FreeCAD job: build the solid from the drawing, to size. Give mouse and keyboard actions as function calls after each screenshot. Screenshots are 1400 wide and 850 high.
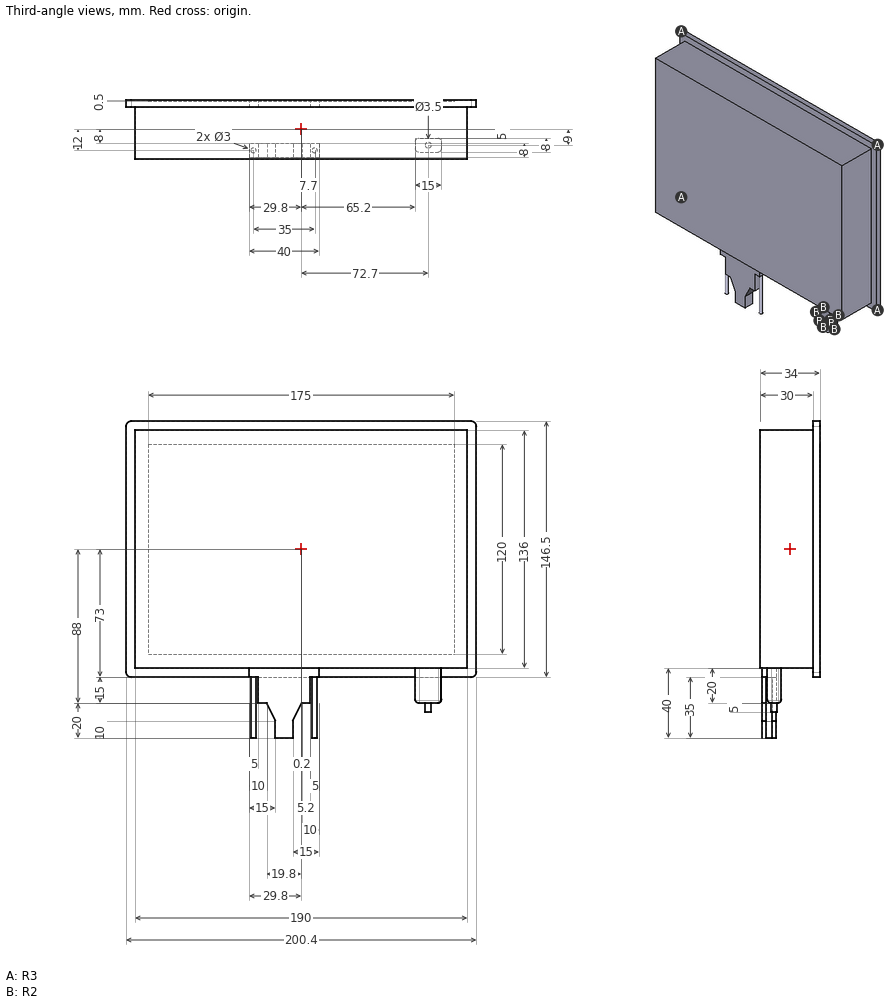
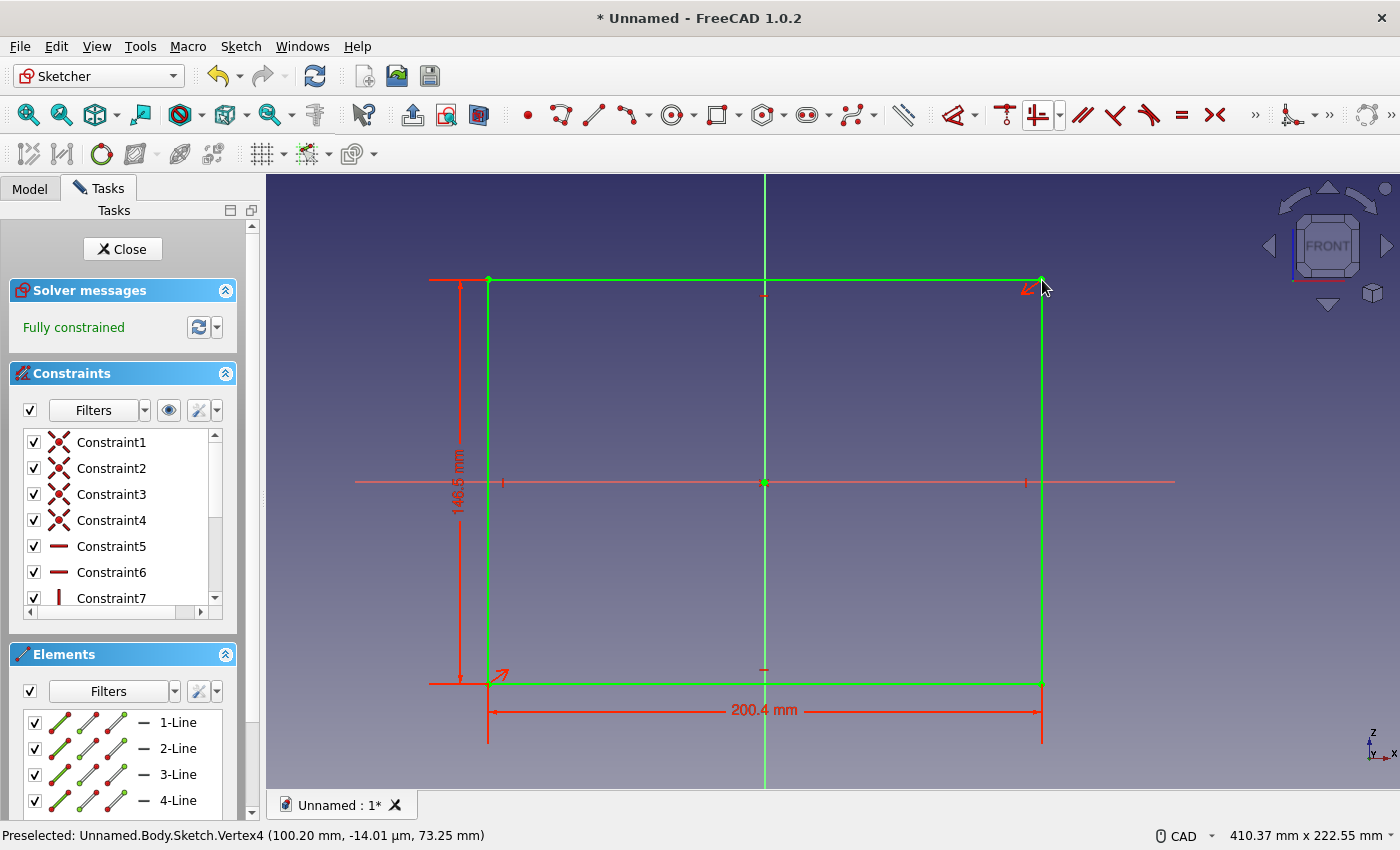
click(123, 249)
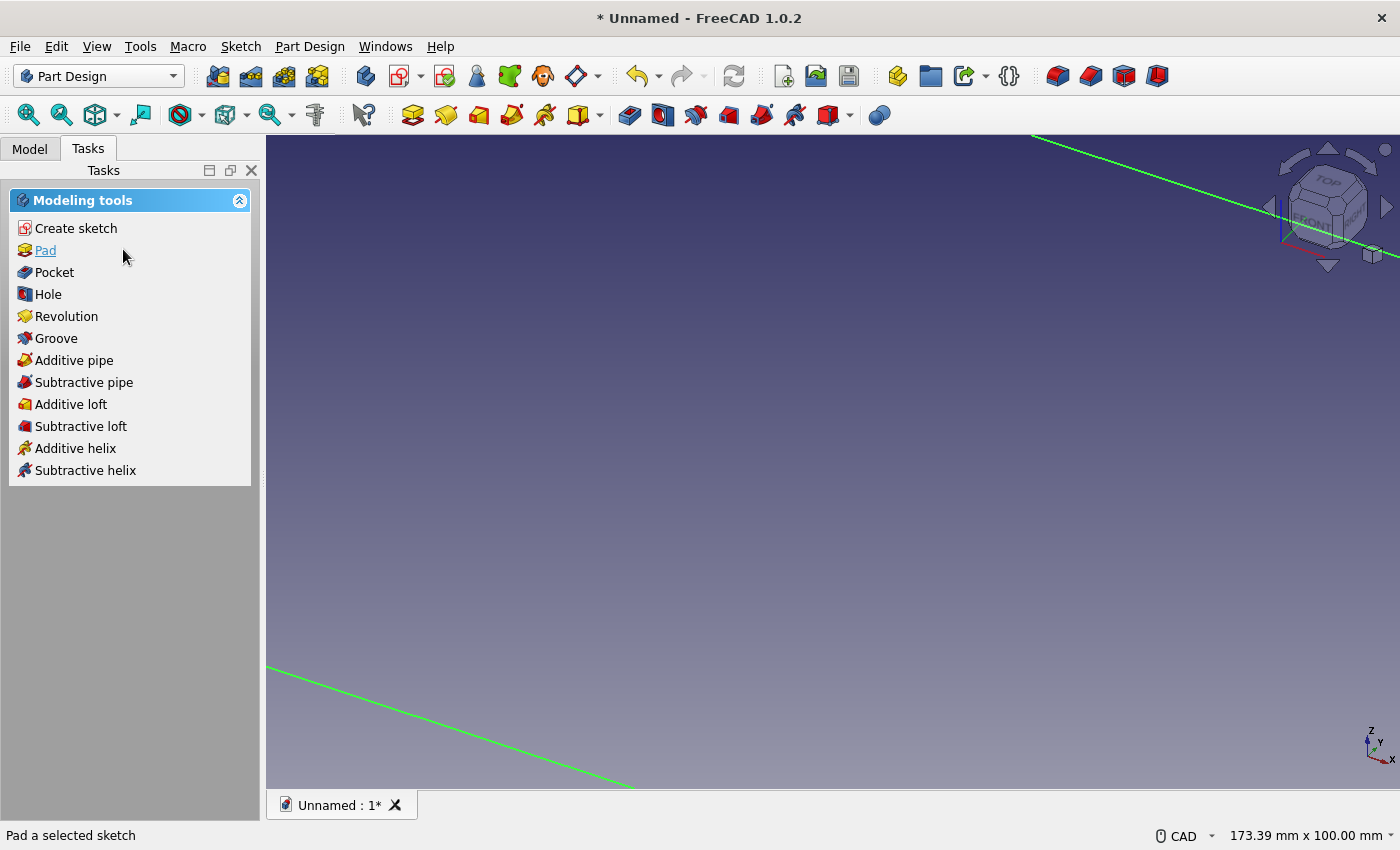
click(413, 116)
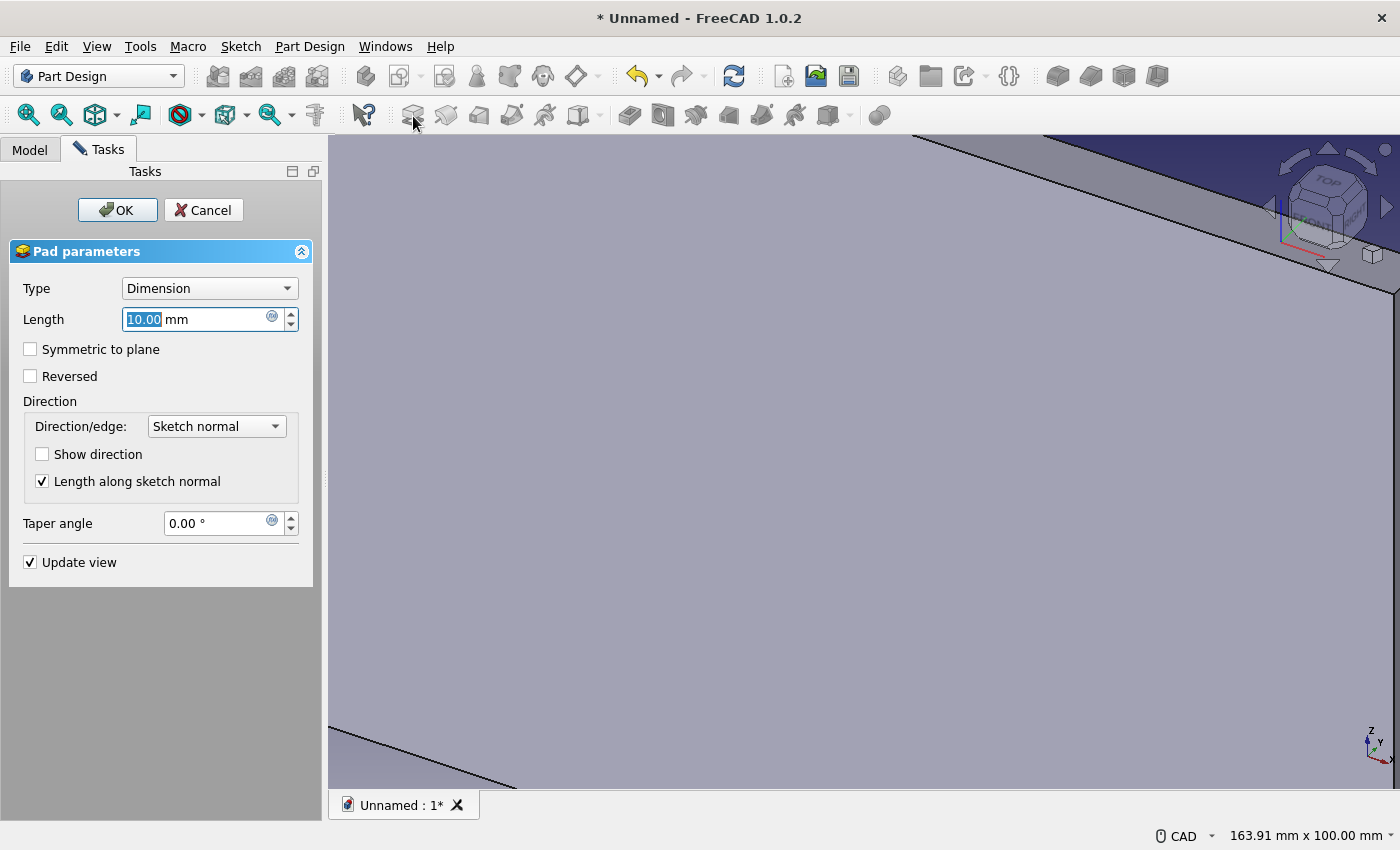
text(34)
key(Tab)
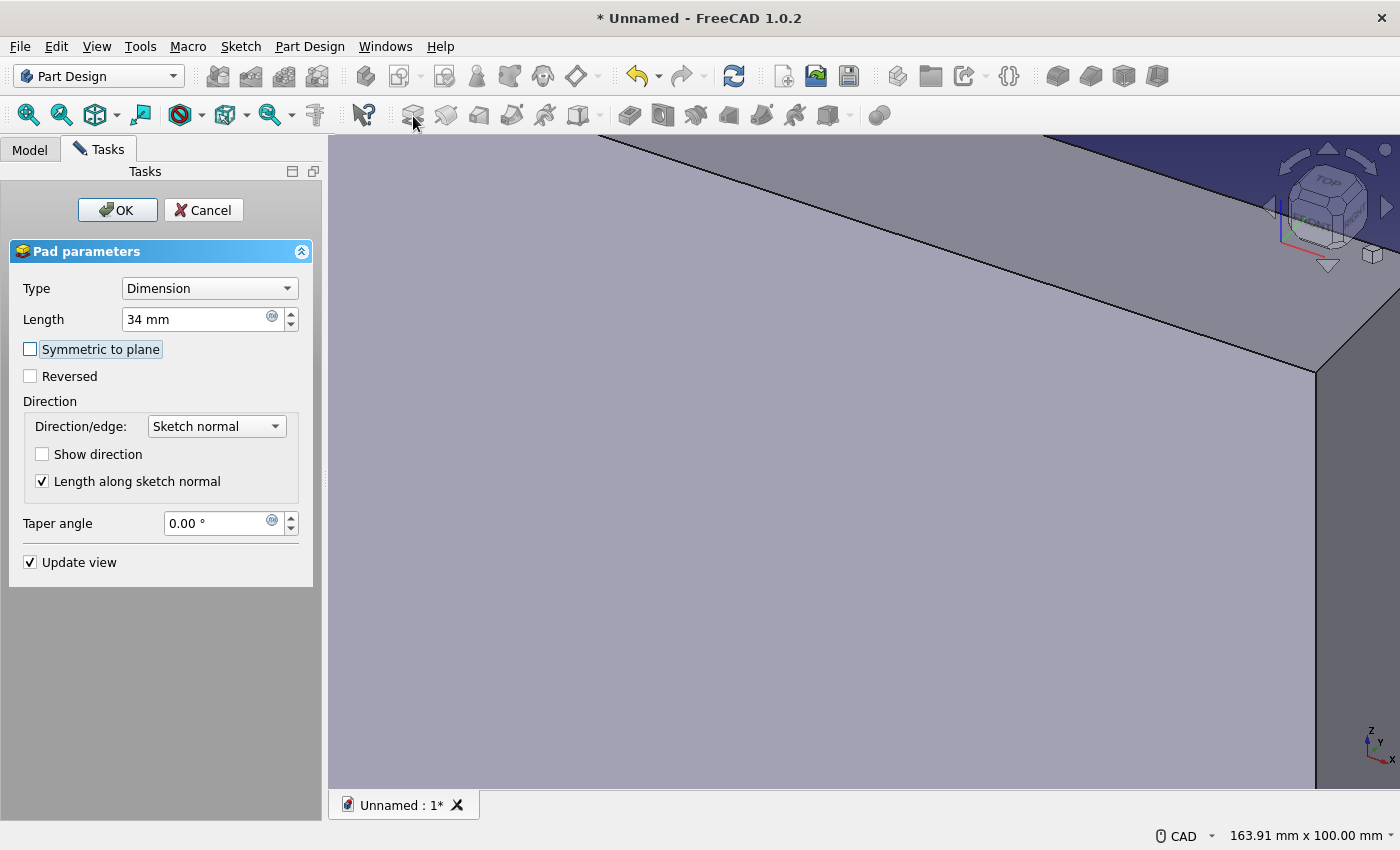
click(31, 349)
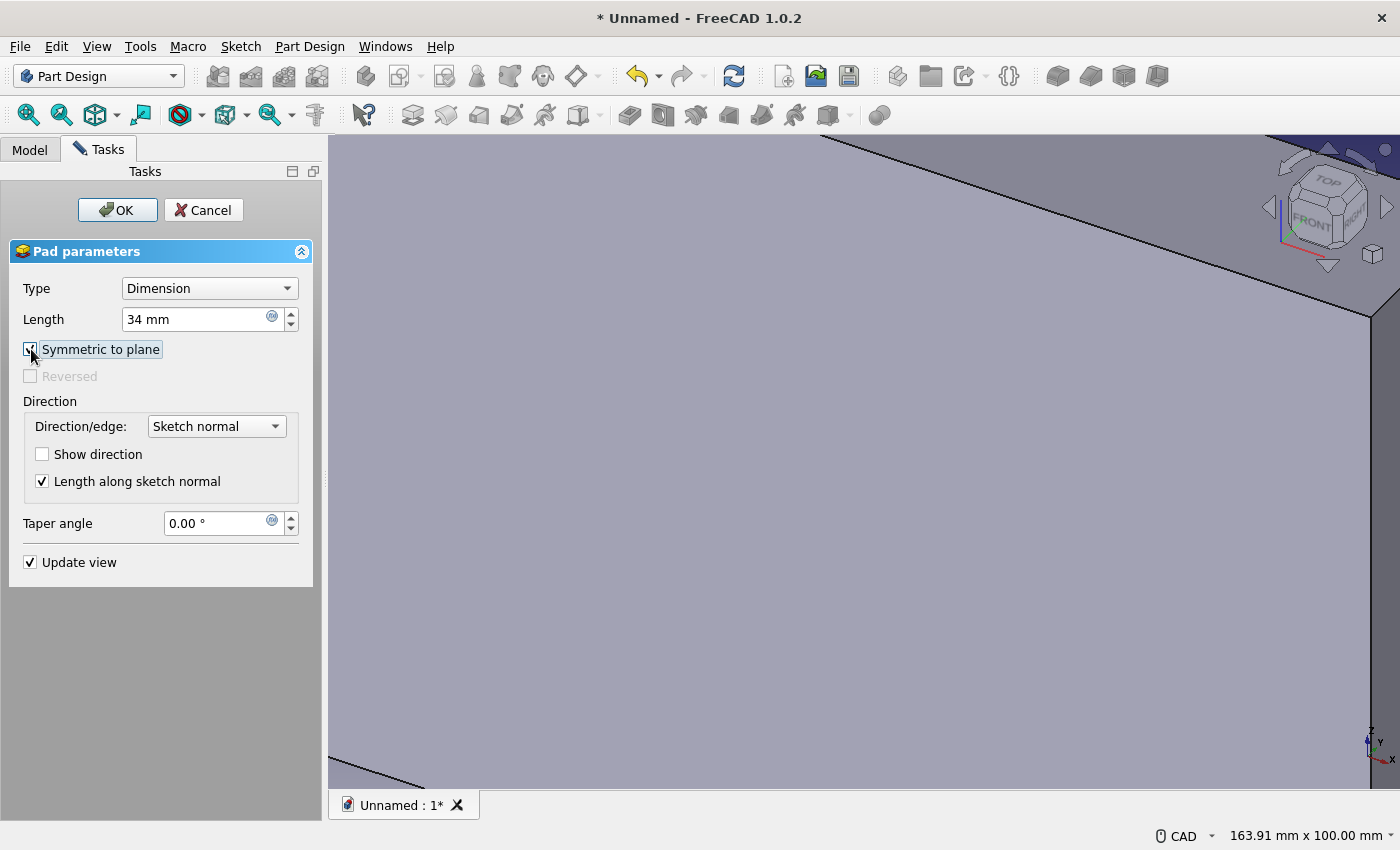
click(118, 210)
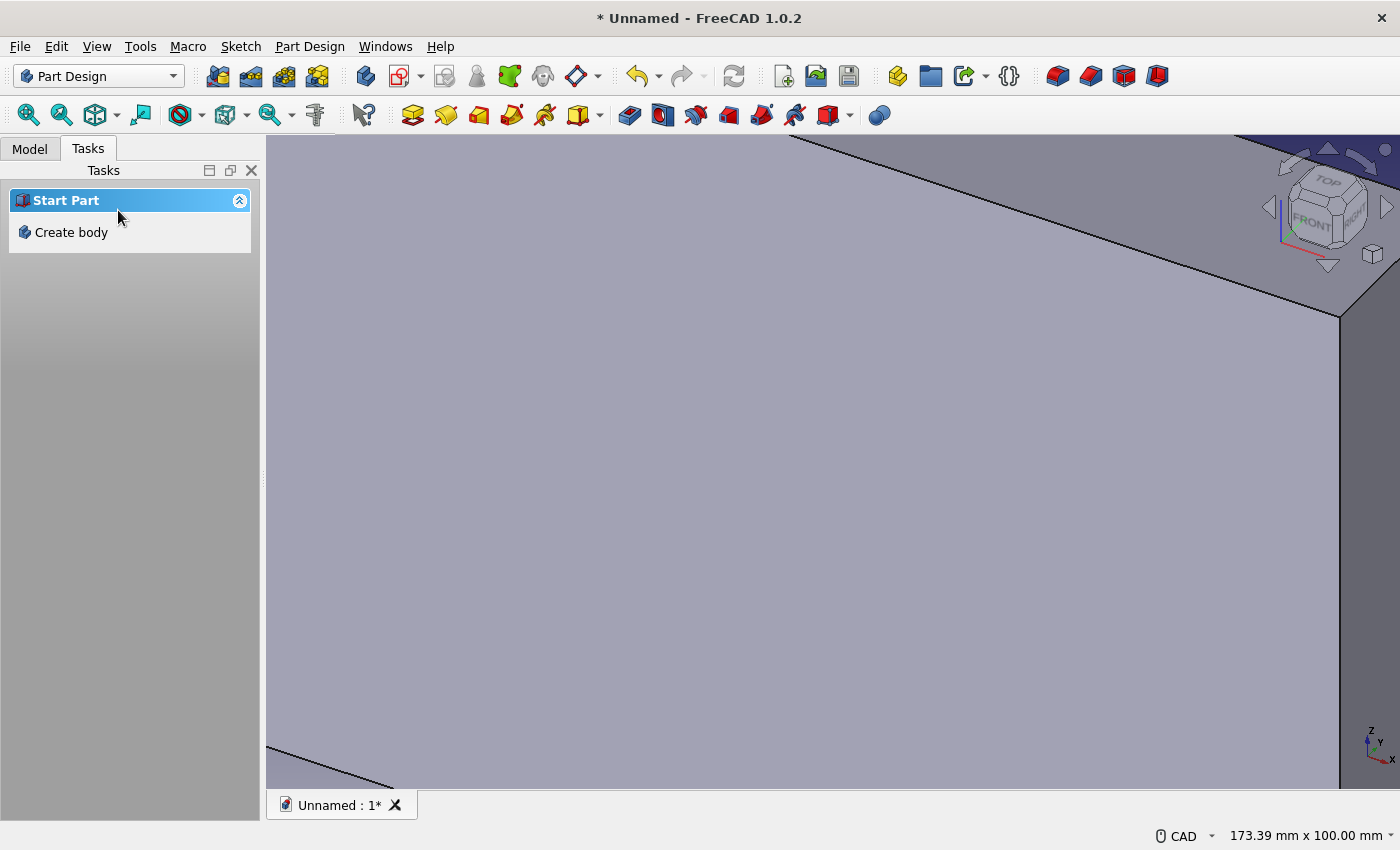
click(29, 116)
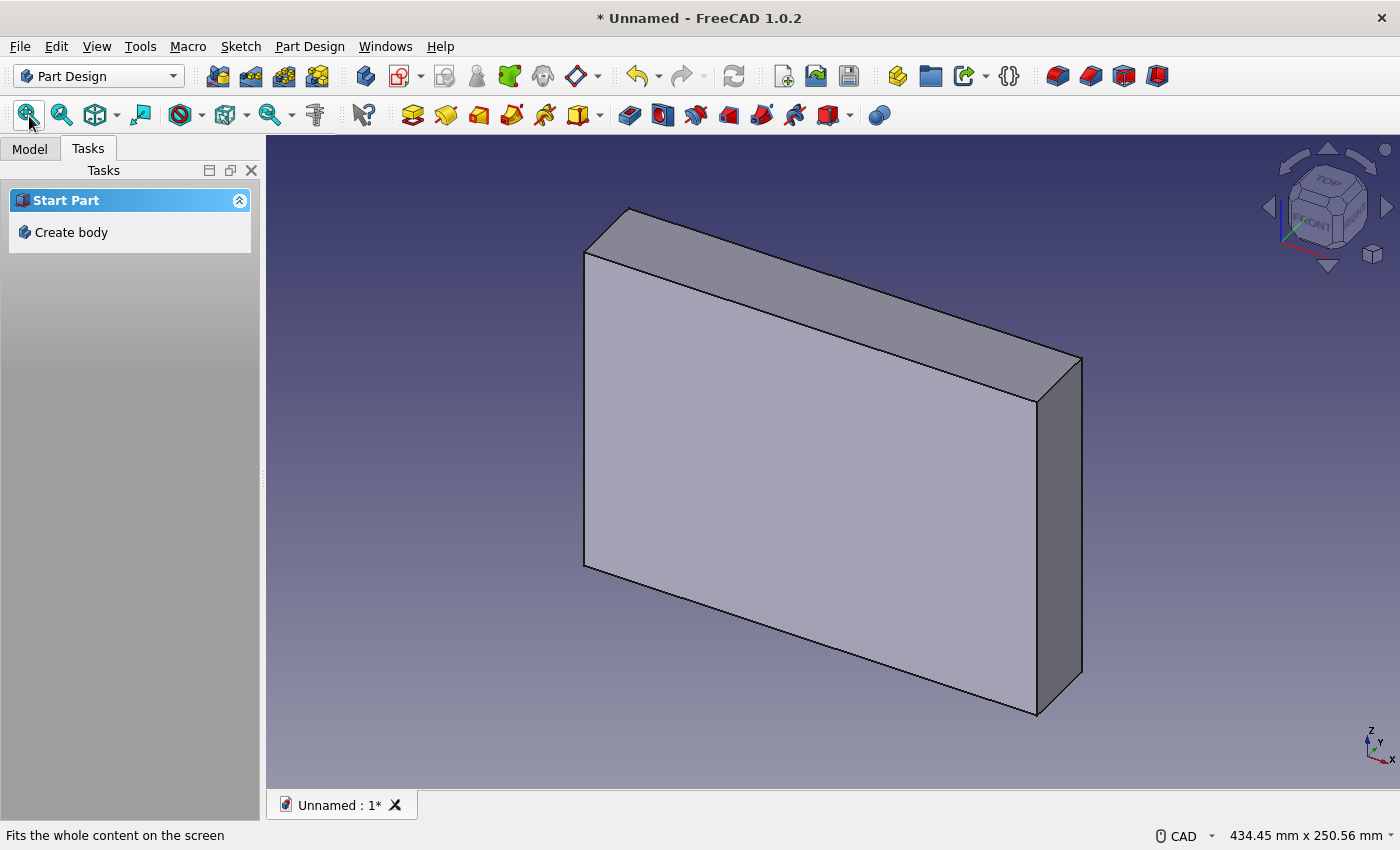
key(4)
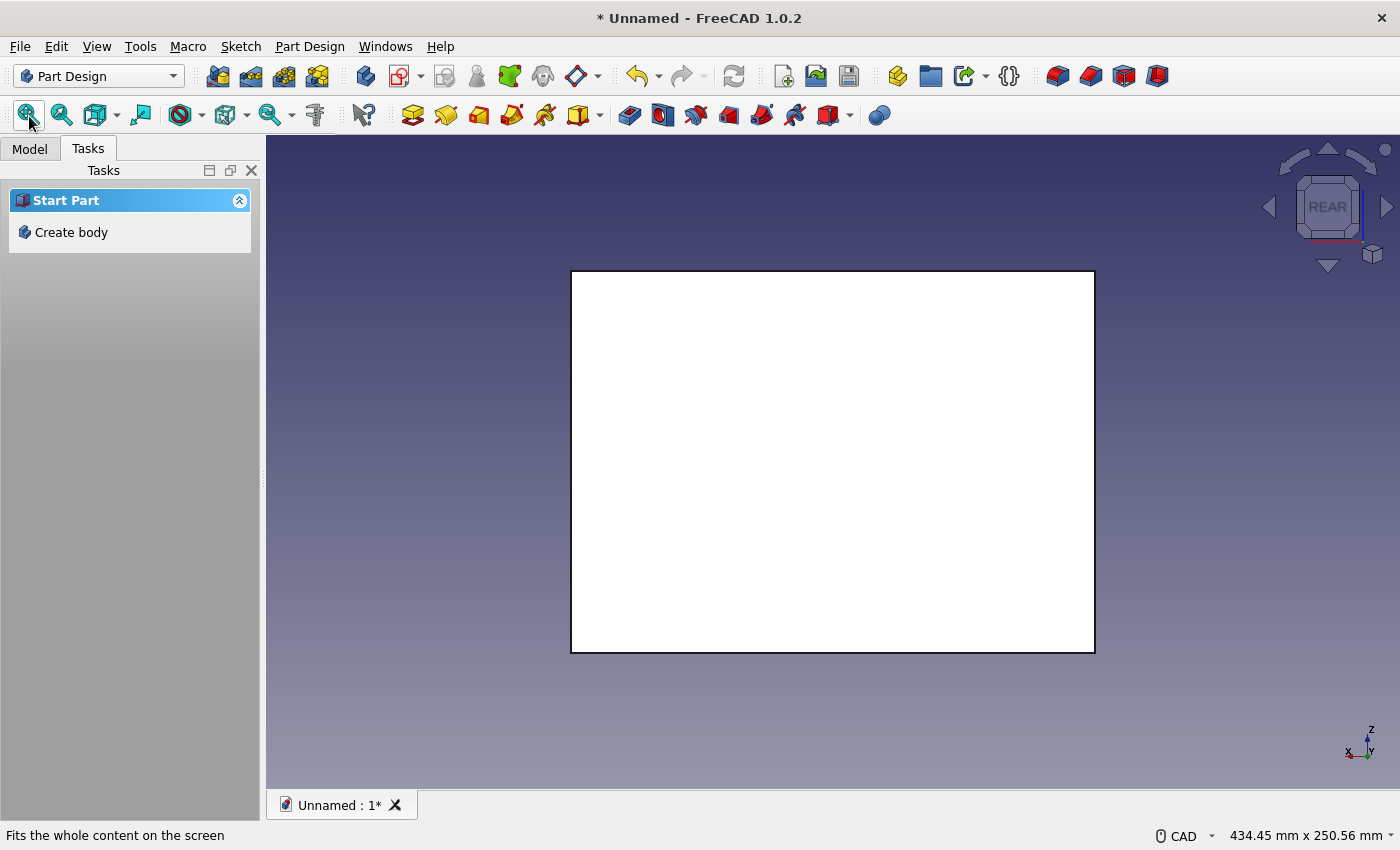
click(833, 461)